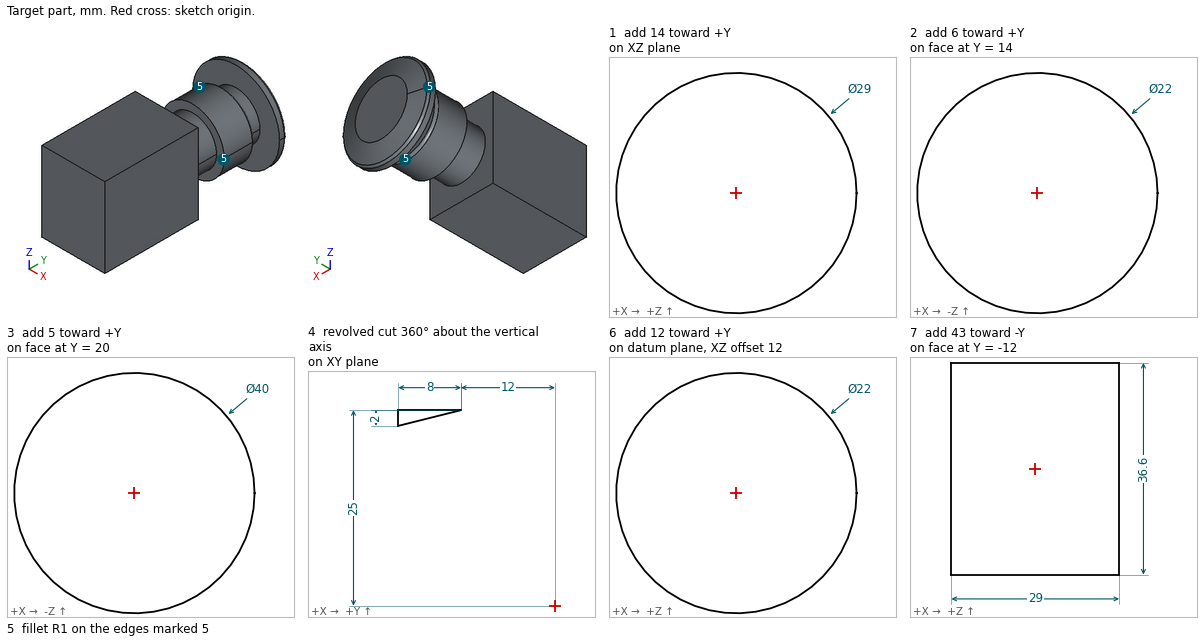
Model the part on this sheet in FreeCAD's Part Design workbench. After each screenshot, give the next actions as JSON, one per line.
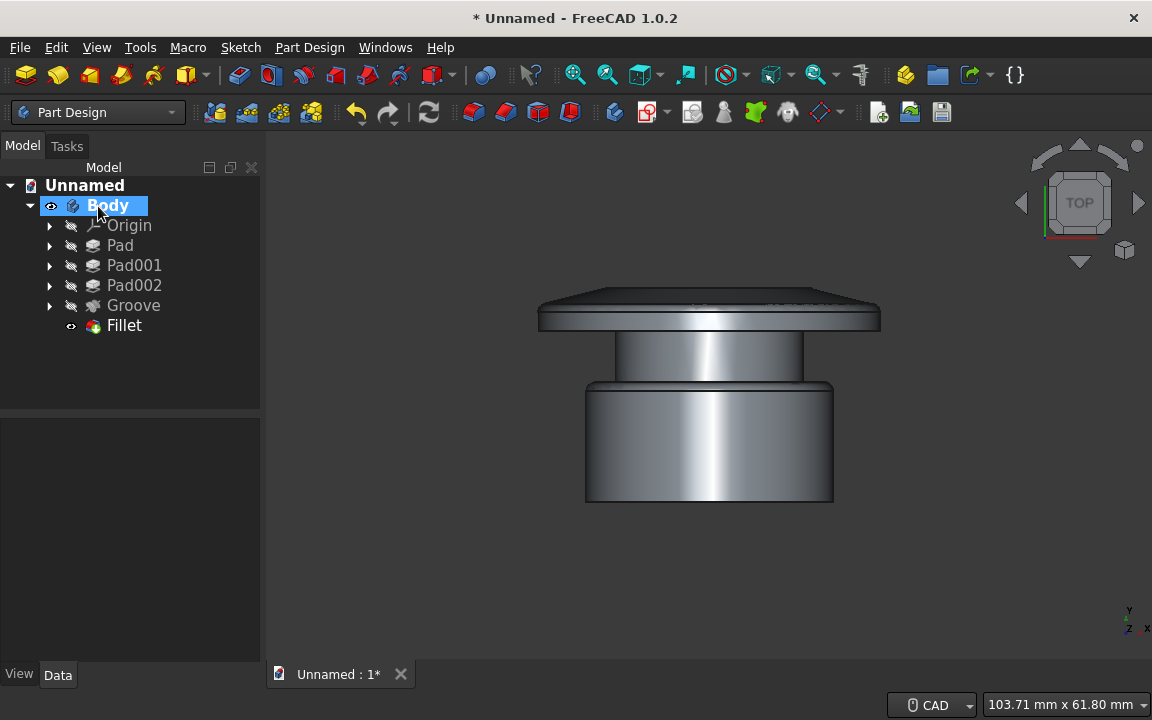
{"action": "key", "text": "v f"}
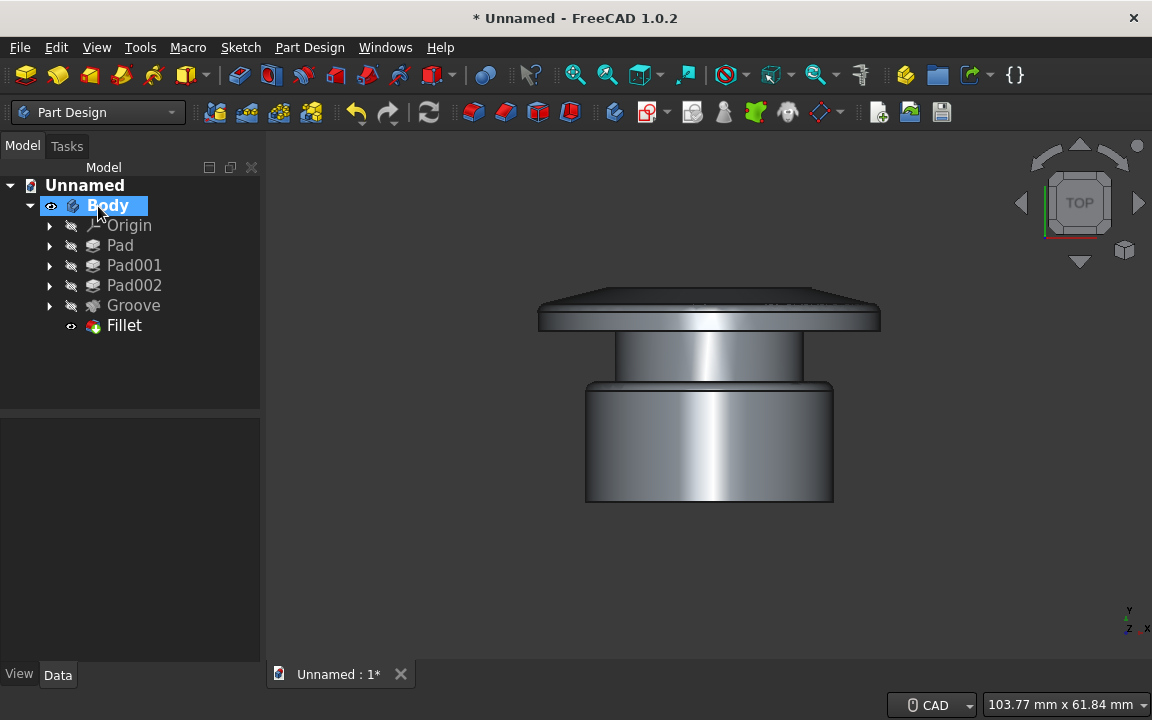
{"action": "left_click", "coordinate": [50, 226]}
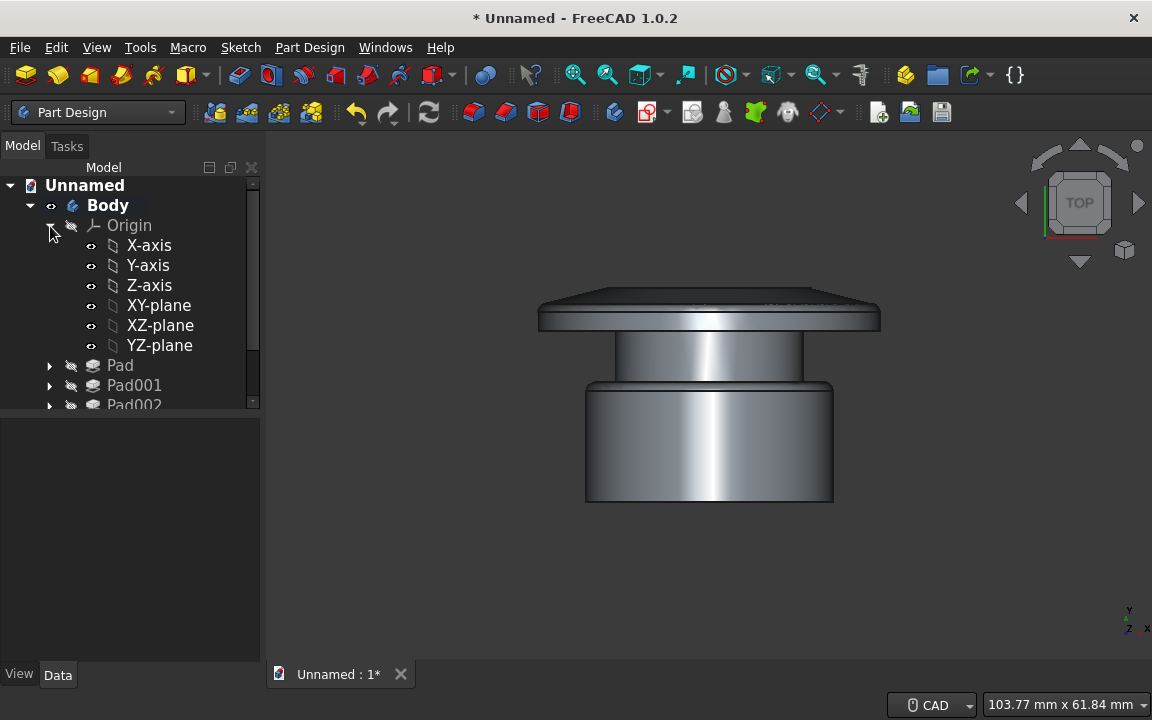
{"action": "left_click", "coordinate": [136, 326]}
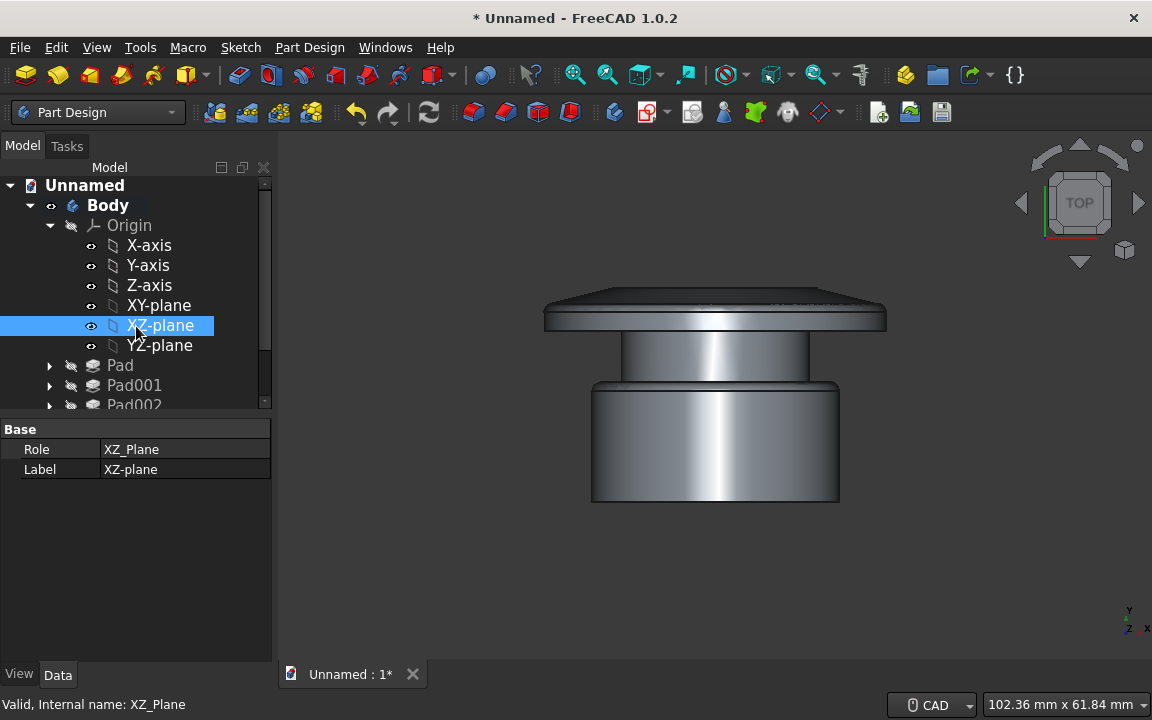
{"action": "left_click", "coordinate": [820, 112]}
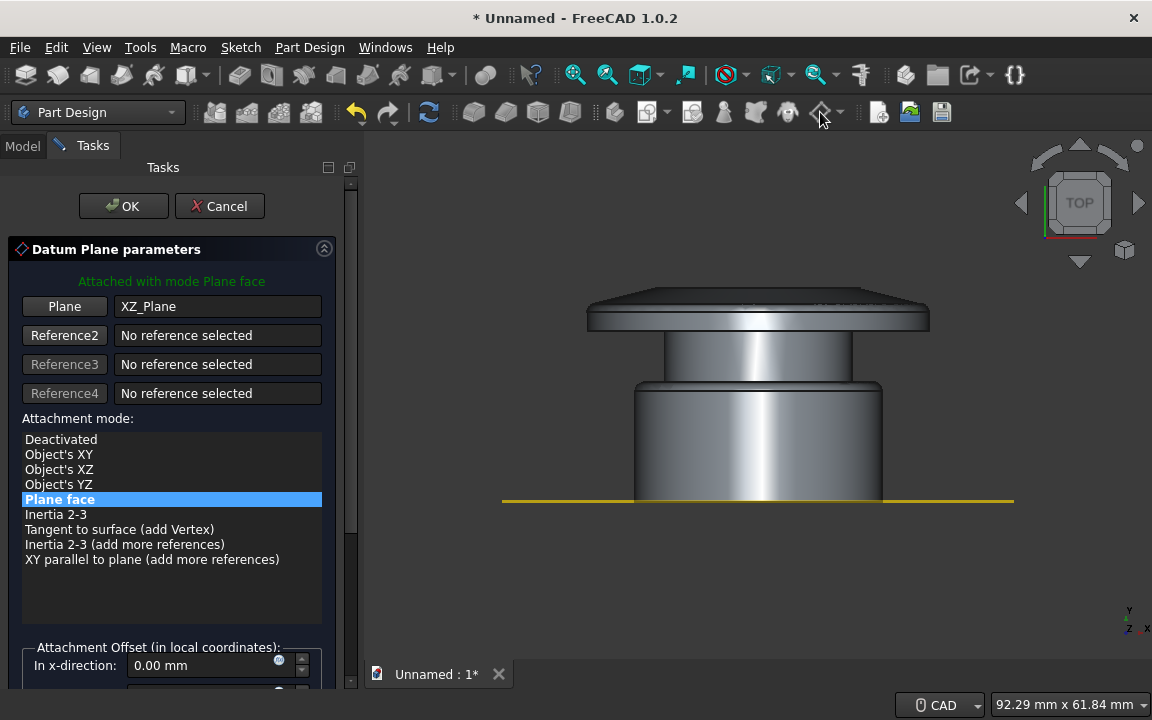
{"action": "scroll", "coordinate": [351, 432], "scroll_direction": "down", "scroll_amount": 2}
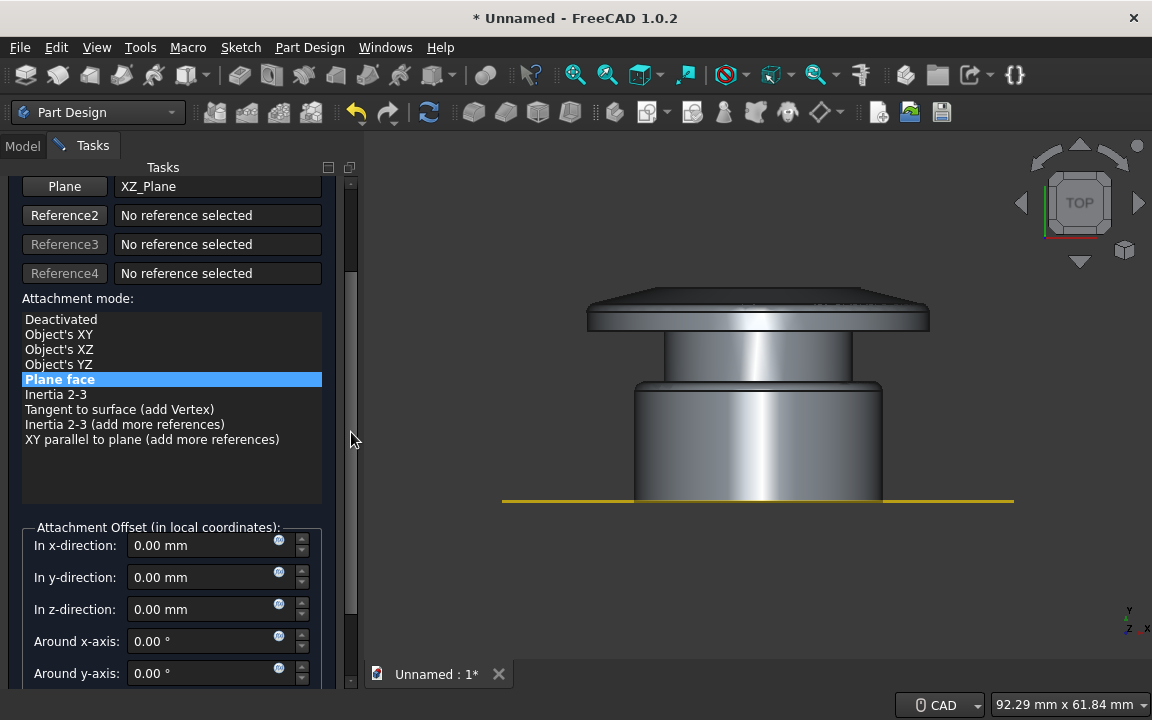
{"action": "triple_click", "coordinate": [210, 609]}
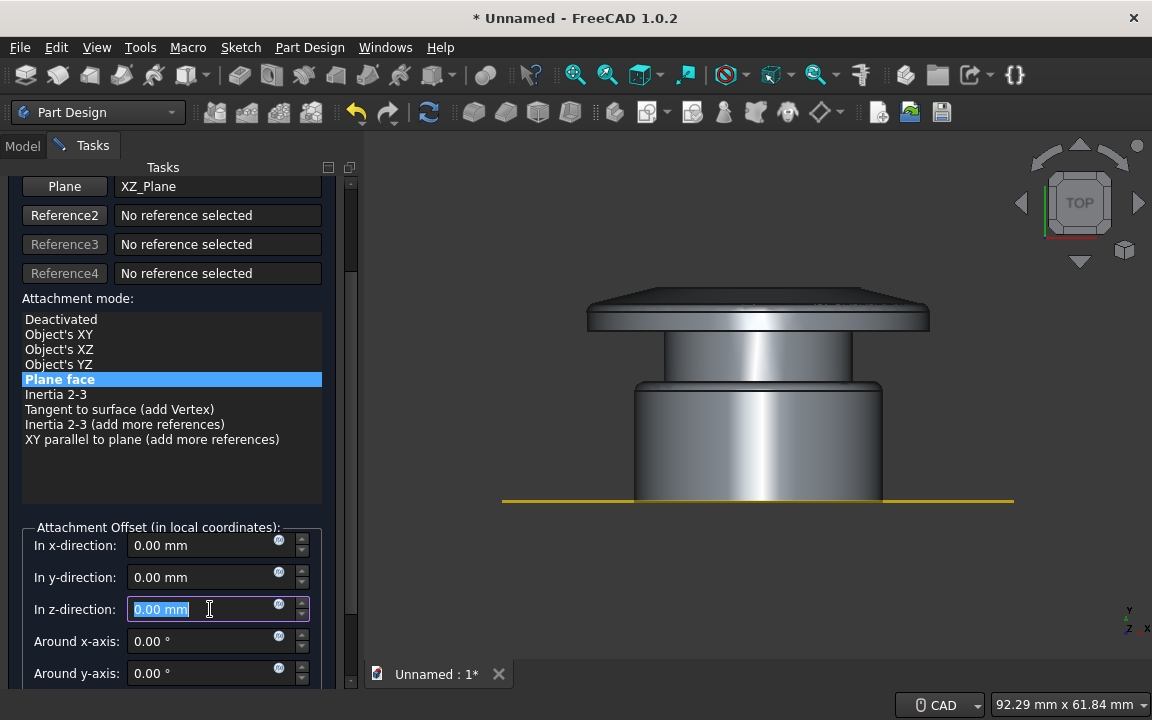
{"action": "type", "text": "12"}
{"action": "key", "text": "Tab"}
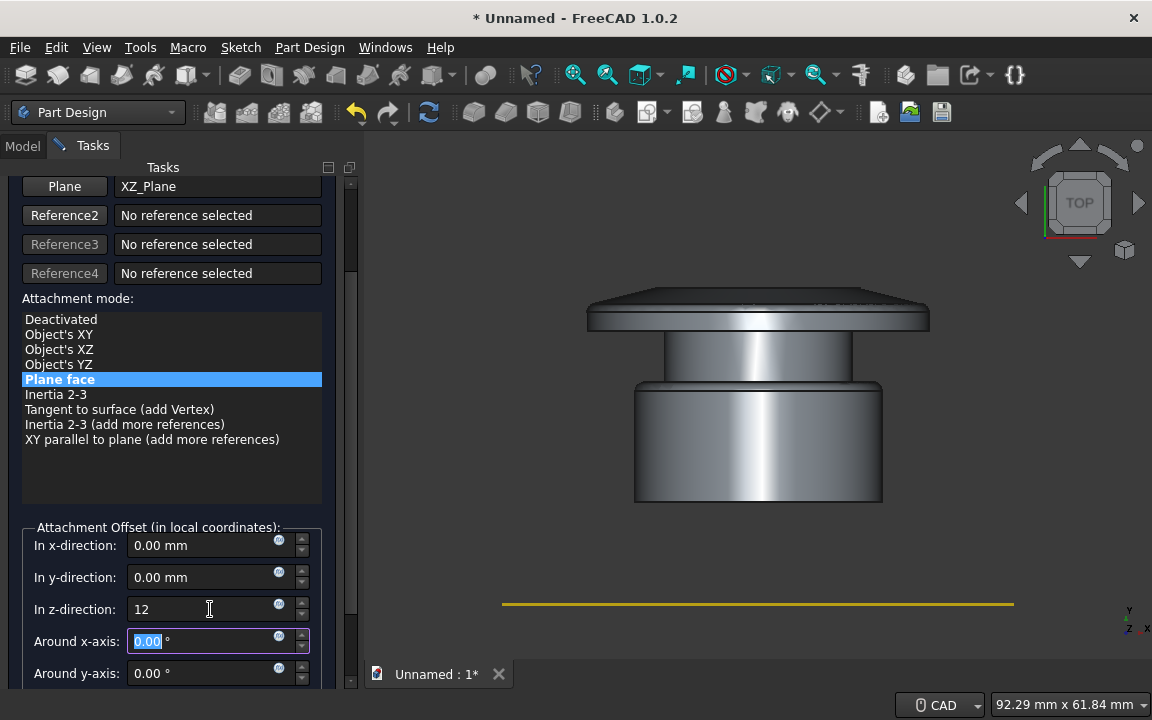
{"action": "scroll", "coordinate": [351, 432], "scroll_direction": "up", "scroll_amount": 3}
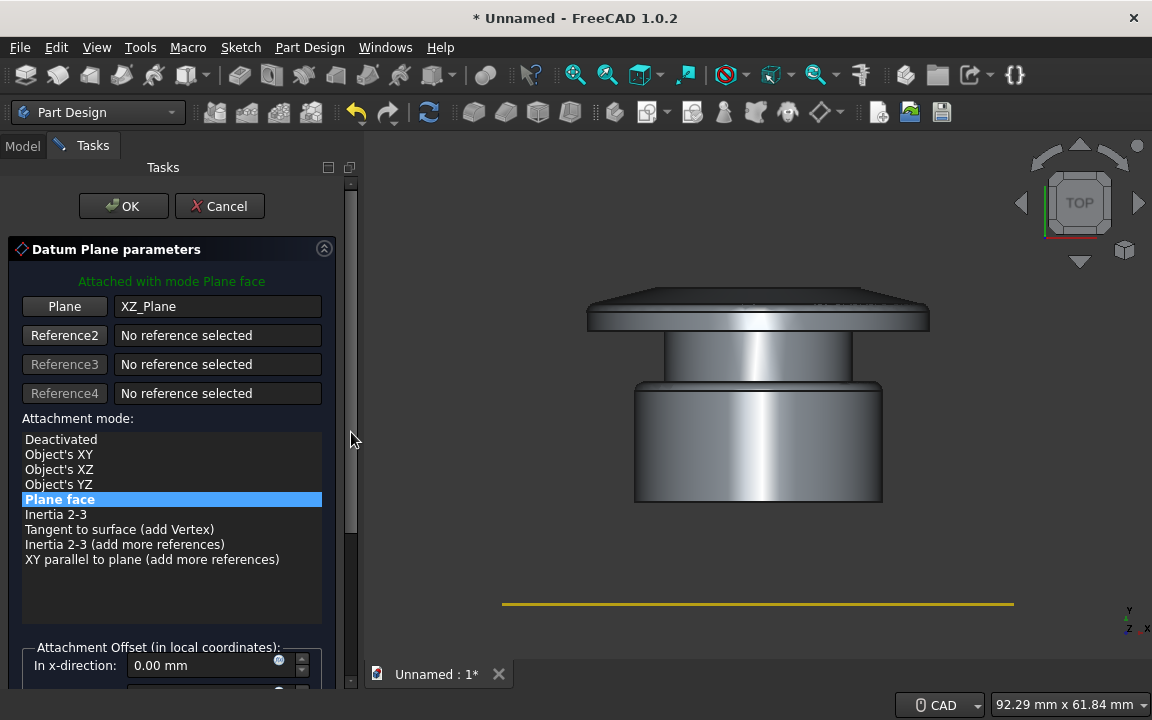
{"action": "left_click", "coordinate": [124, 206]}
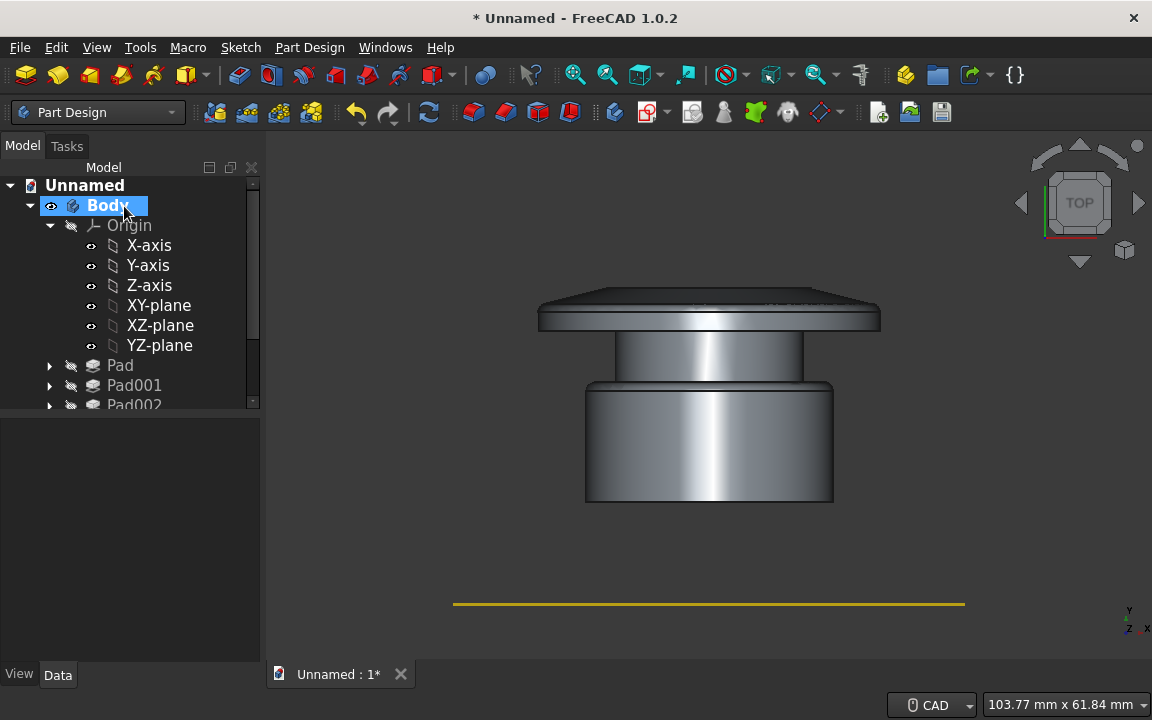
{"action": "scroll", "coordinate": [100, 301], "scroll_direction": "down", "scroll_amount": 3}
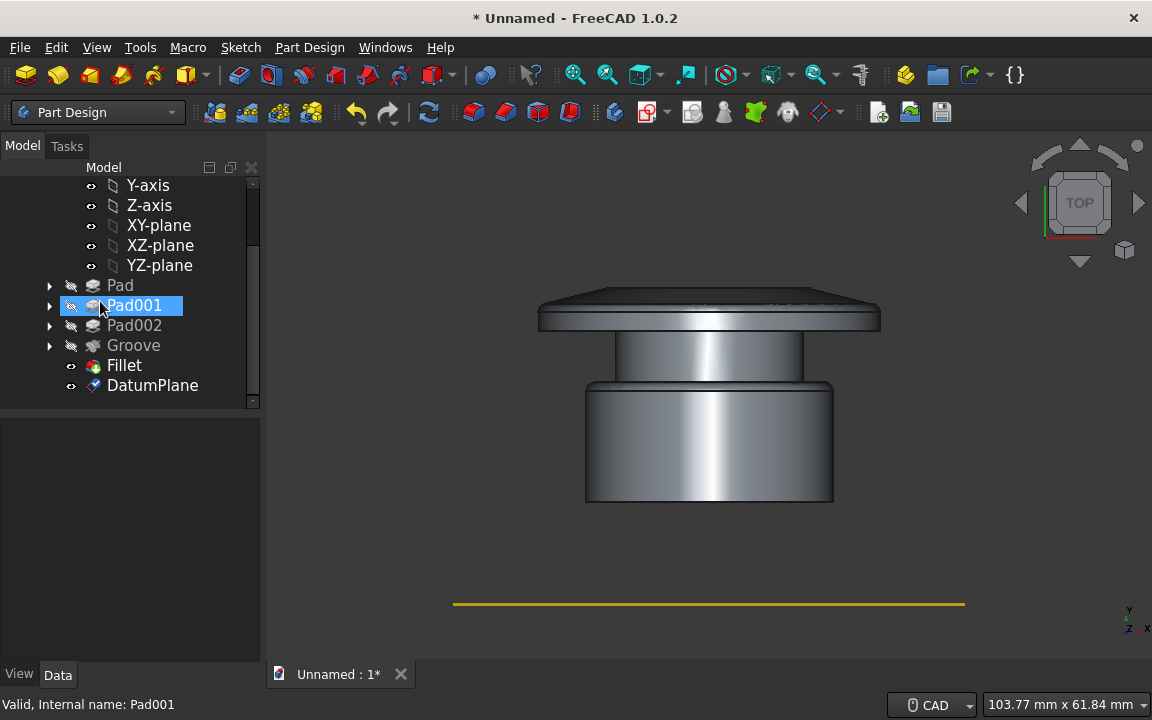
{"action": "left_click", "coordinate": [116, 386]}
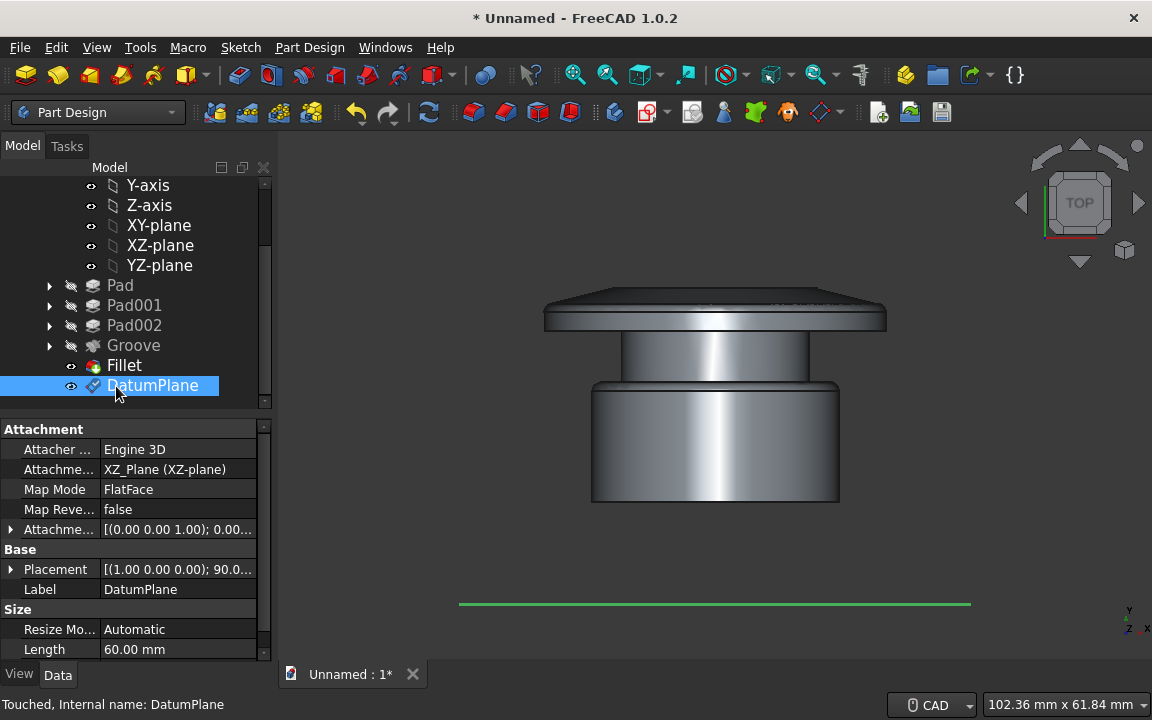
{"action": "left_click", "coordinate": [648, 112]}